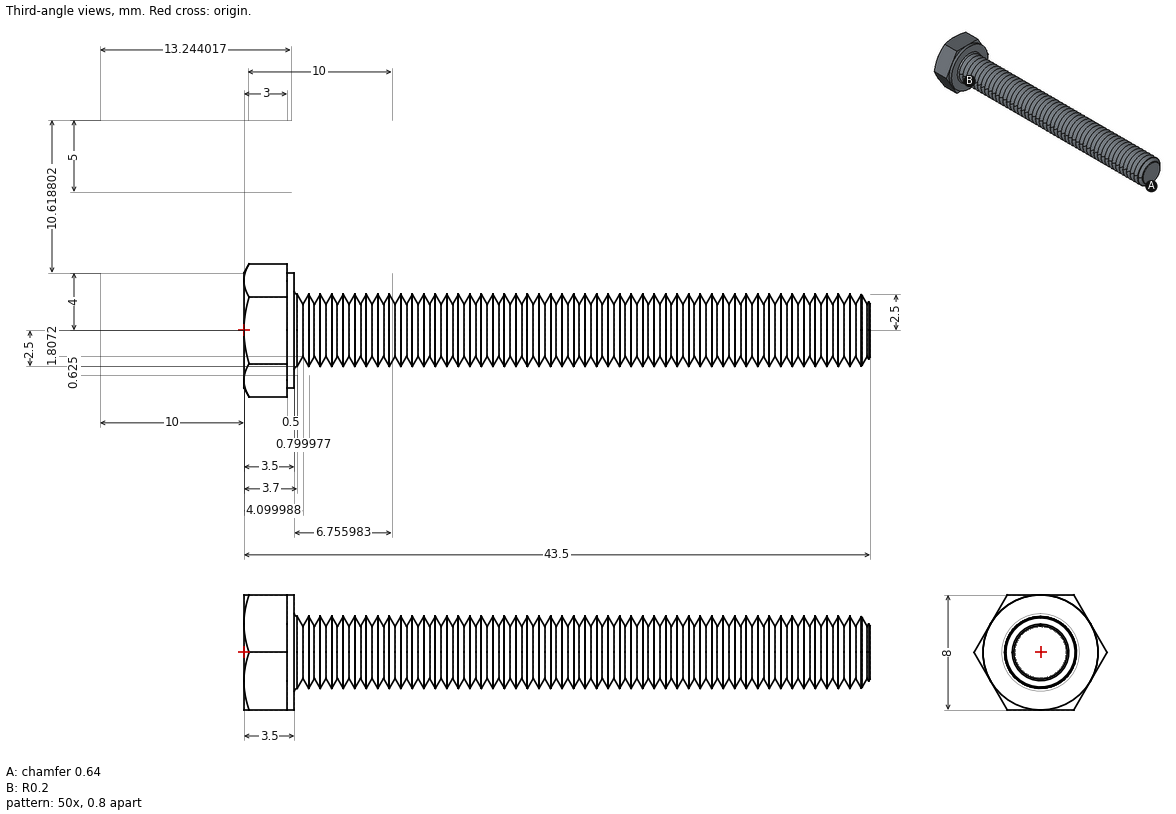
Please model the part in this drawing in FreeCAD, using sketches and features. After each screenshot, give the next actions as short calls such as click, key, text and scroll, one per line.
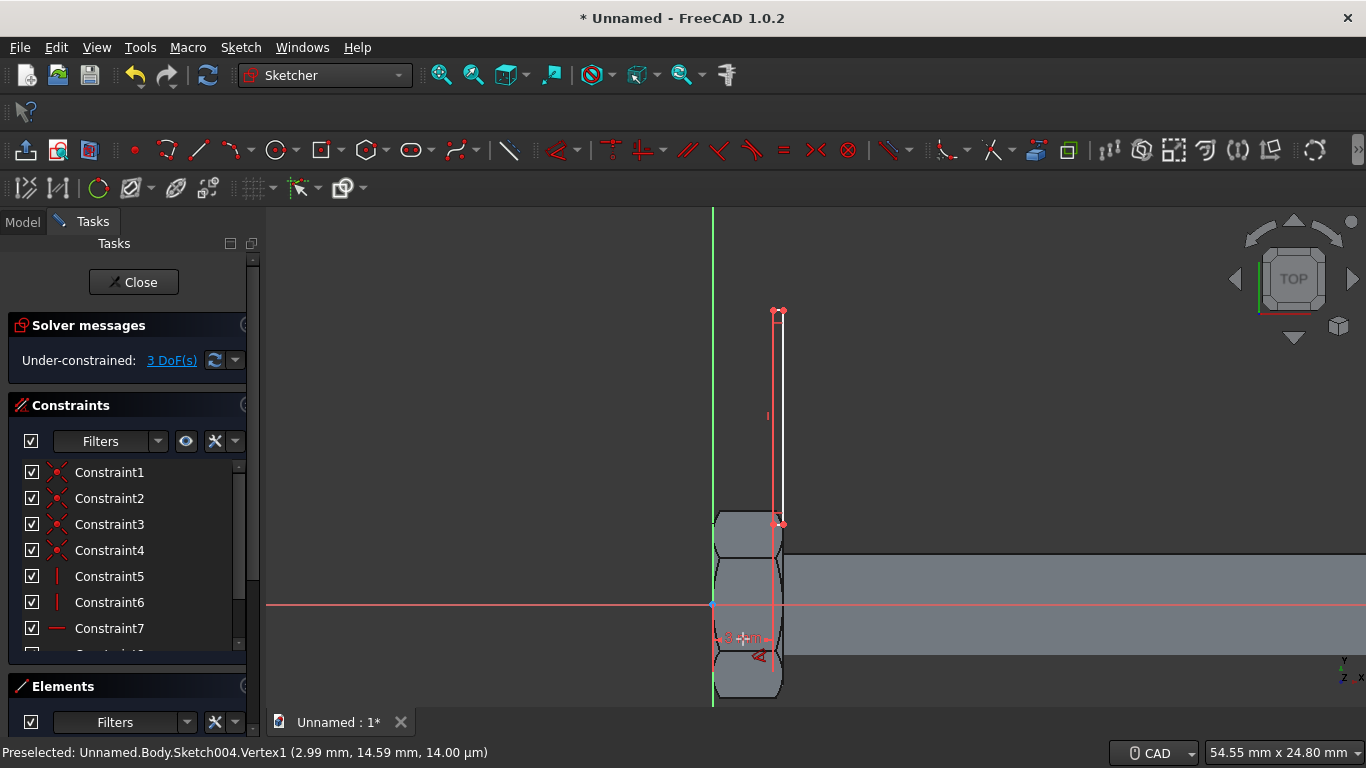
scroll(773, 525, up, 2)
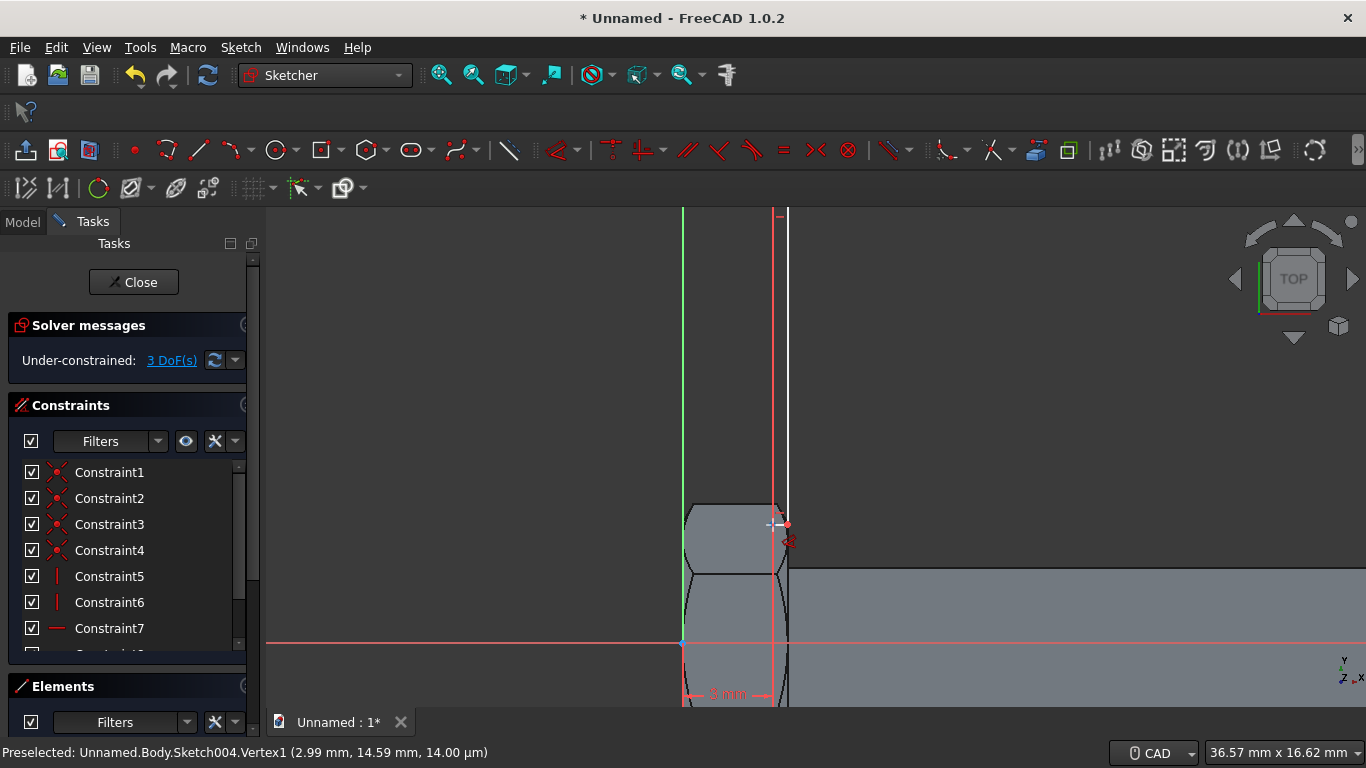
click(773, 525)
click(649, 584)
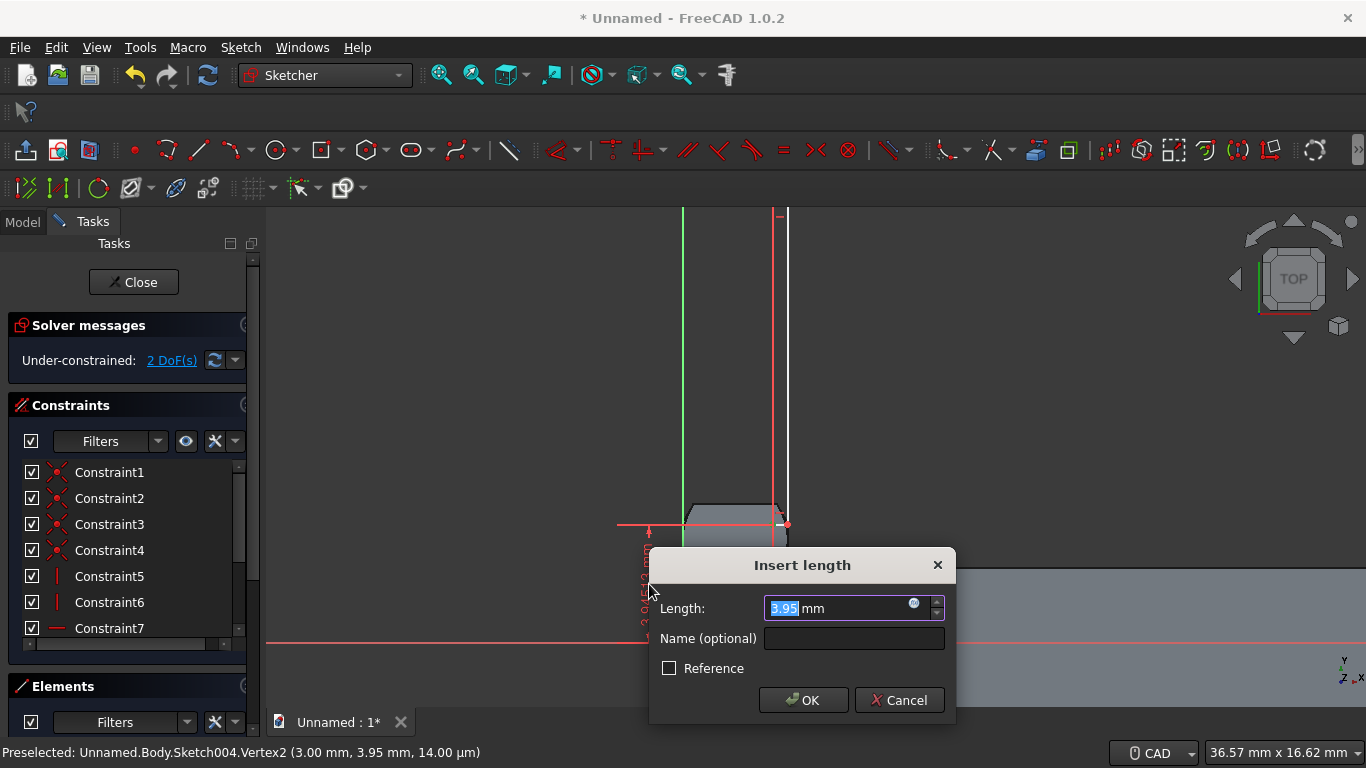
text(4)
key(Return)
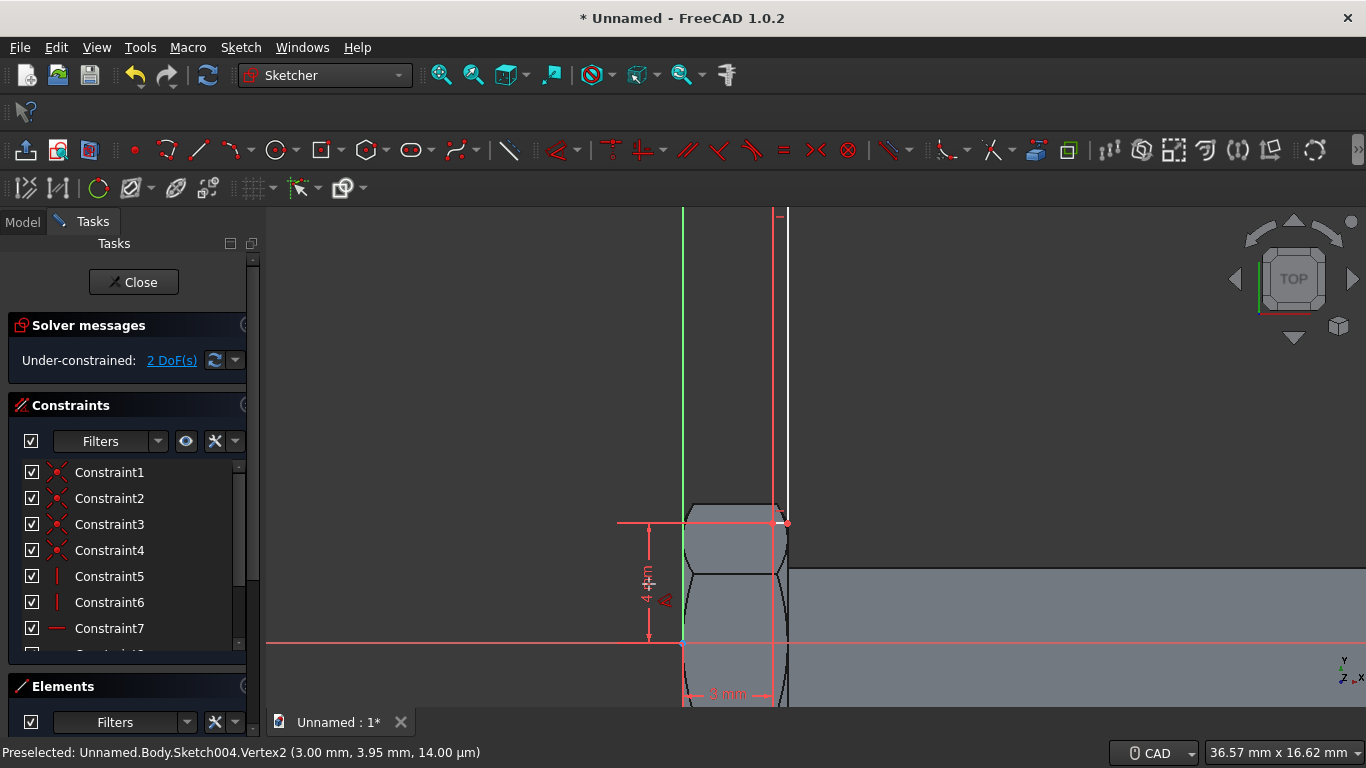
scroll(780, 523, up, 5)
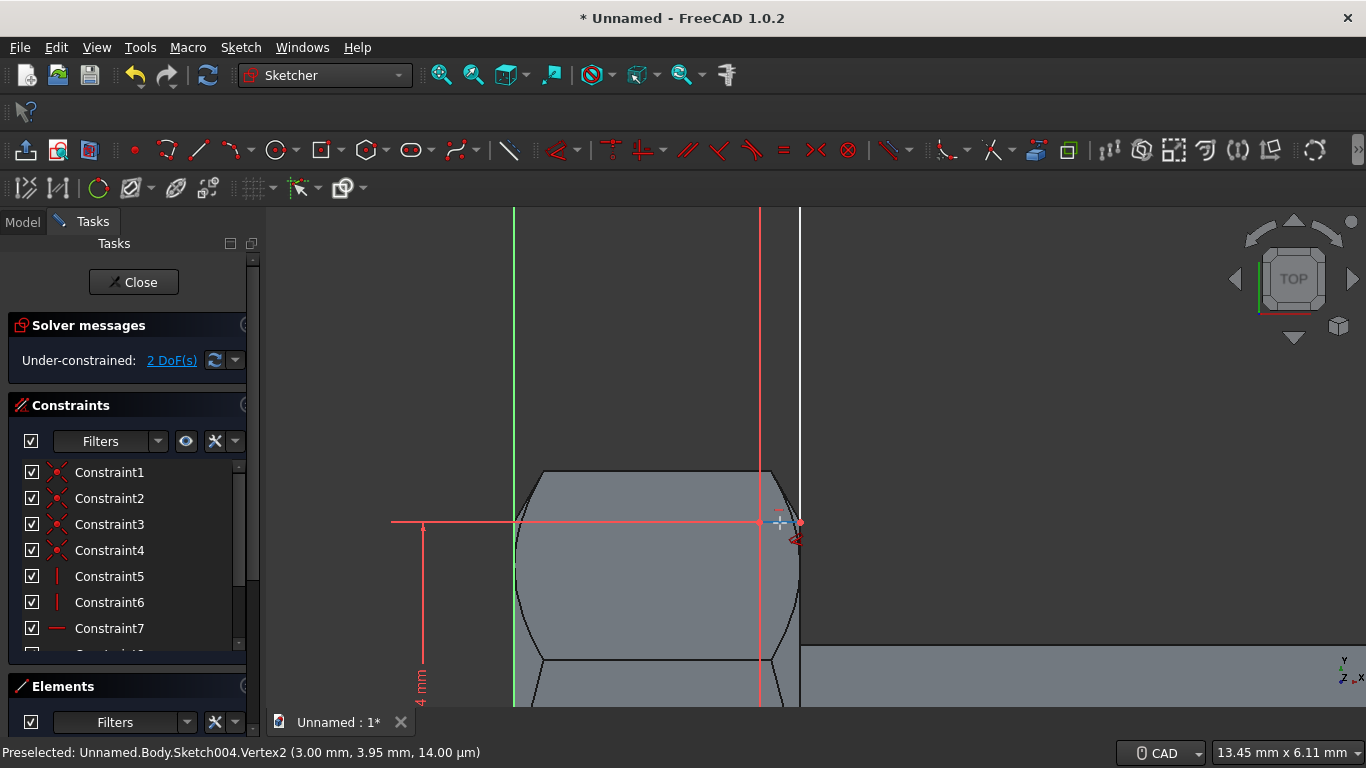
click(780, 522)
click(780, 556)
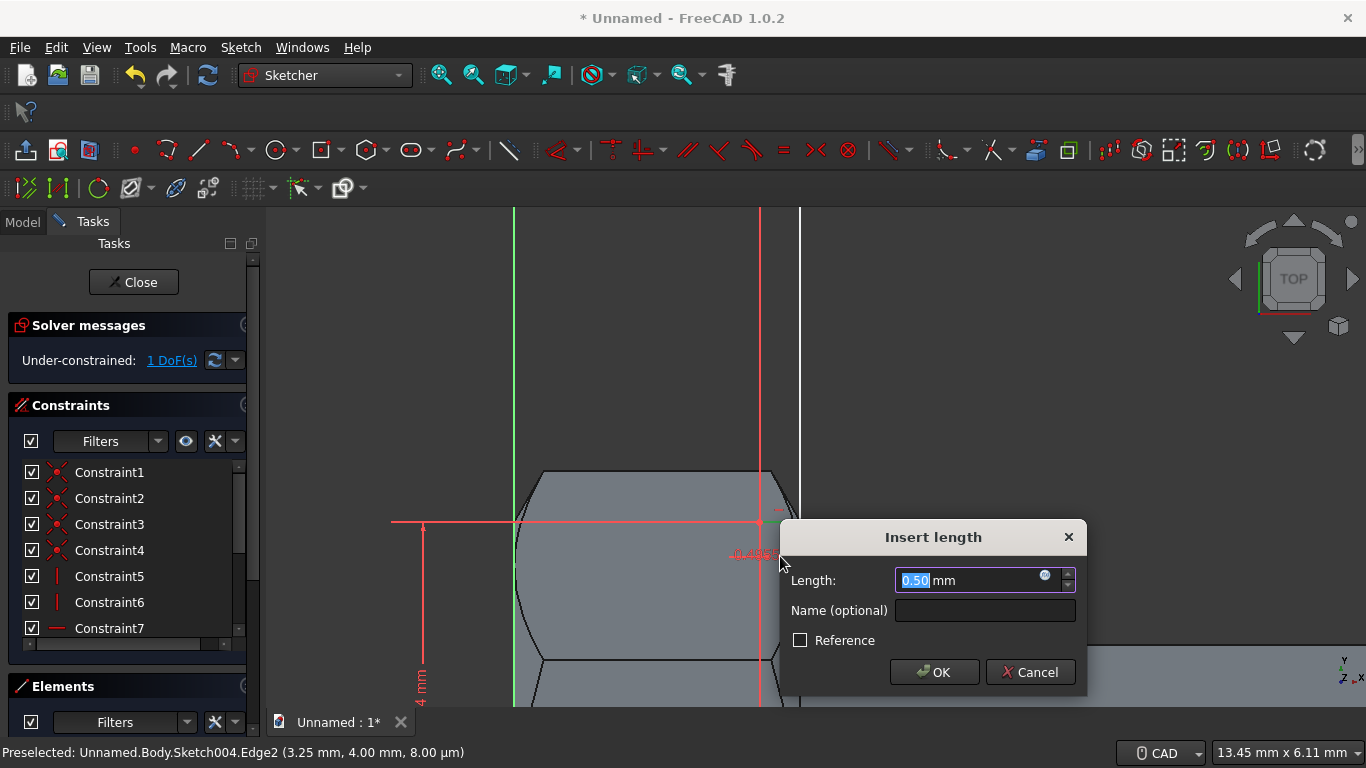
text(0.5)
key(Return)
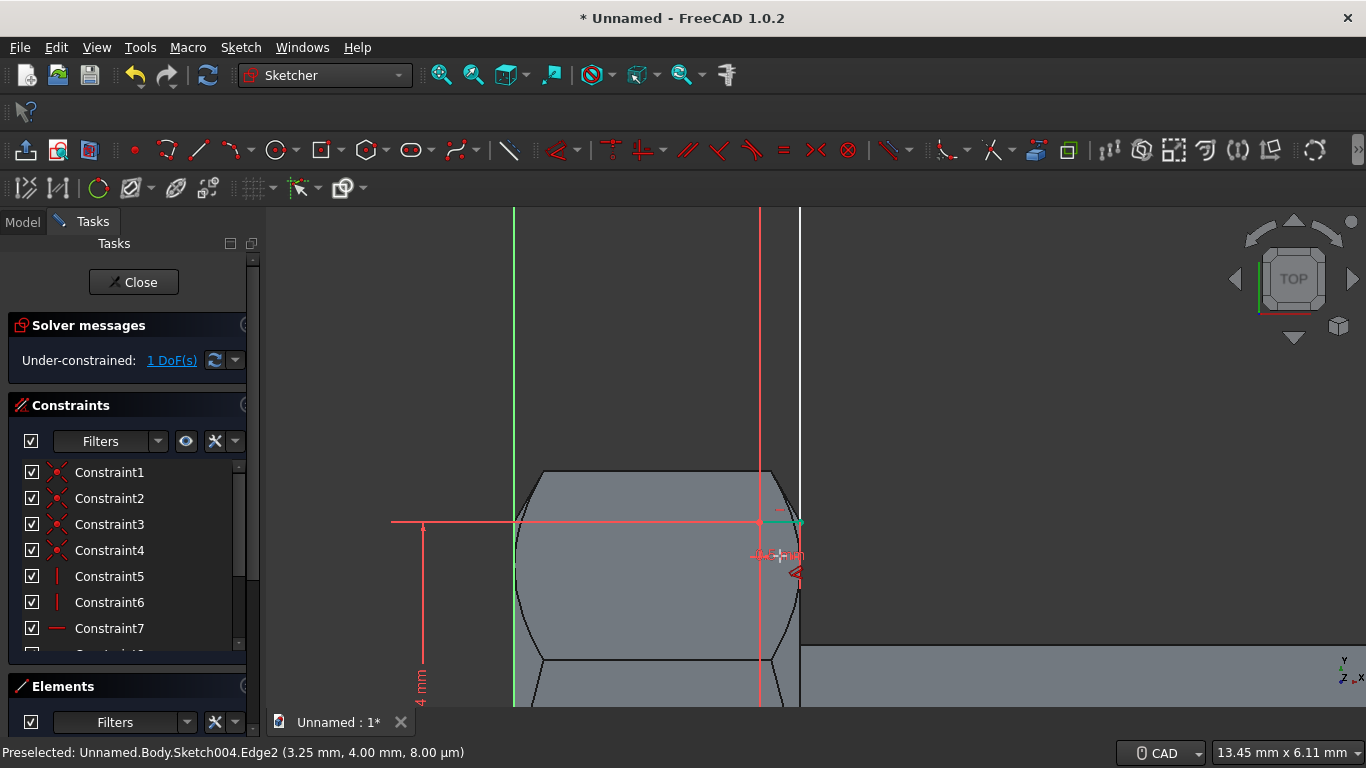
scroll(777, 524, down, 7)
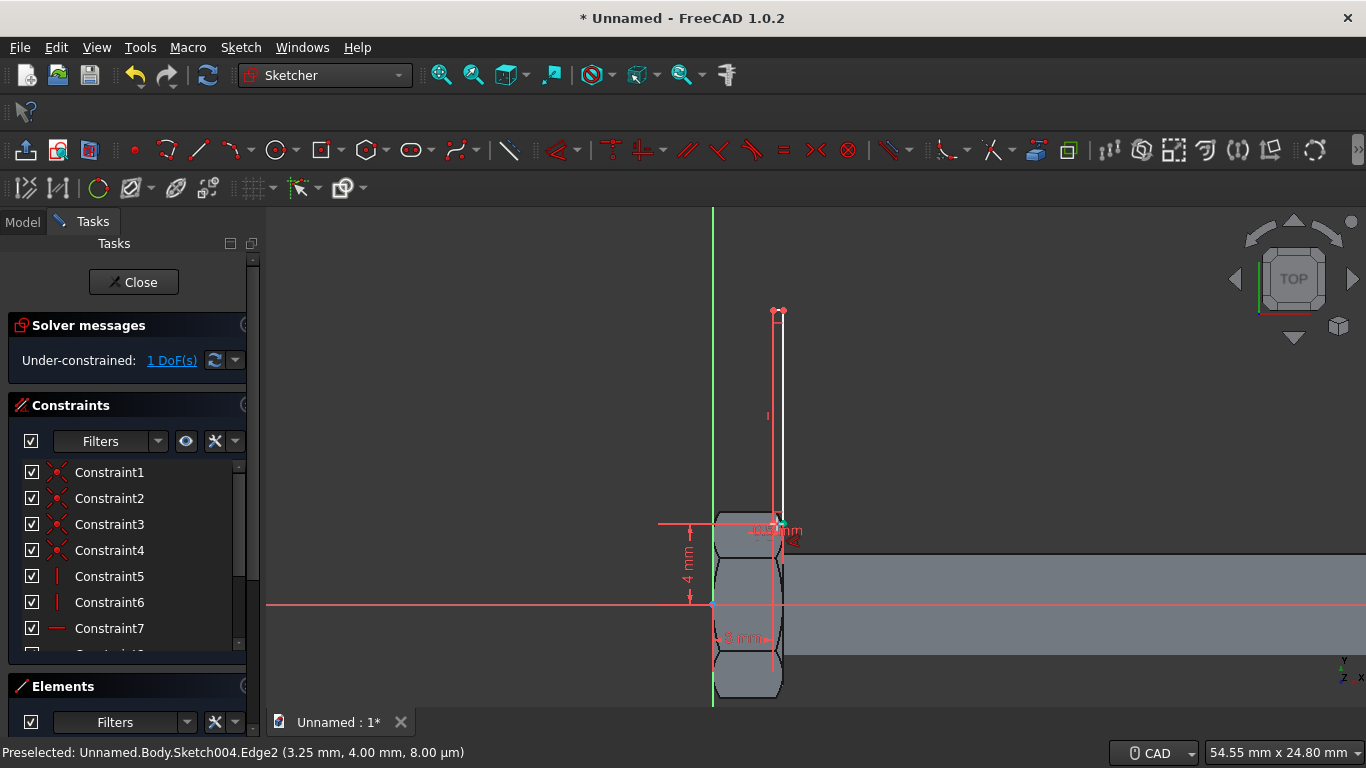
scroll(773, 460, up, 2)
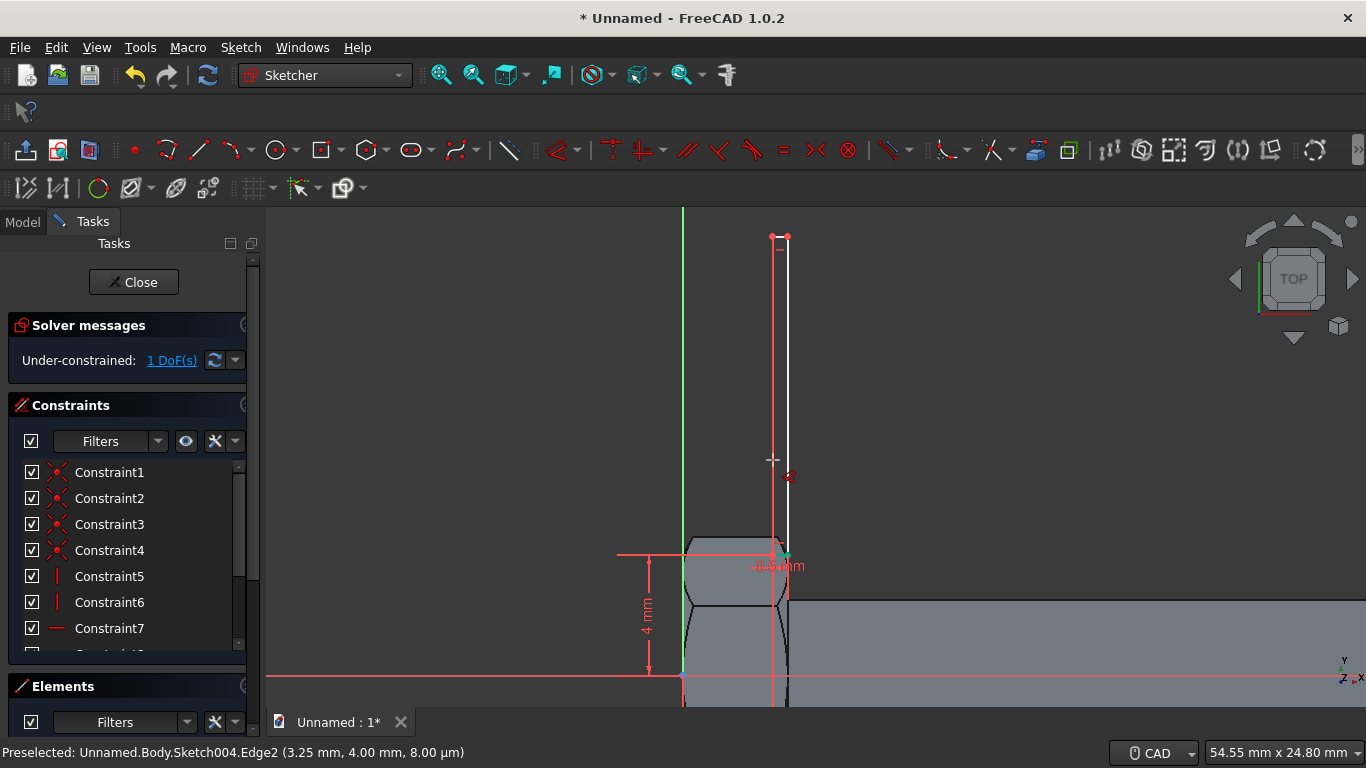
click(773, 460)
click(807, 396)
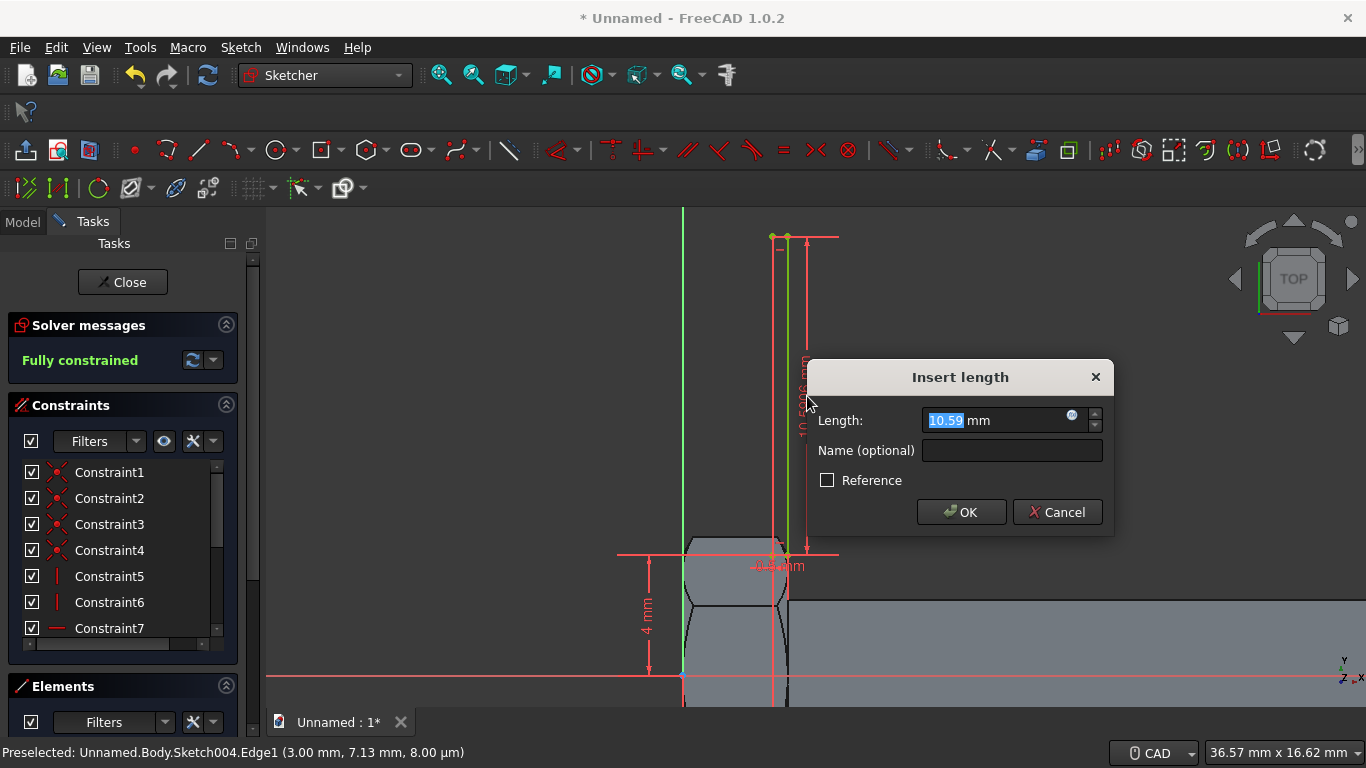
text(10.618802)
key(Return)
key(Escape)